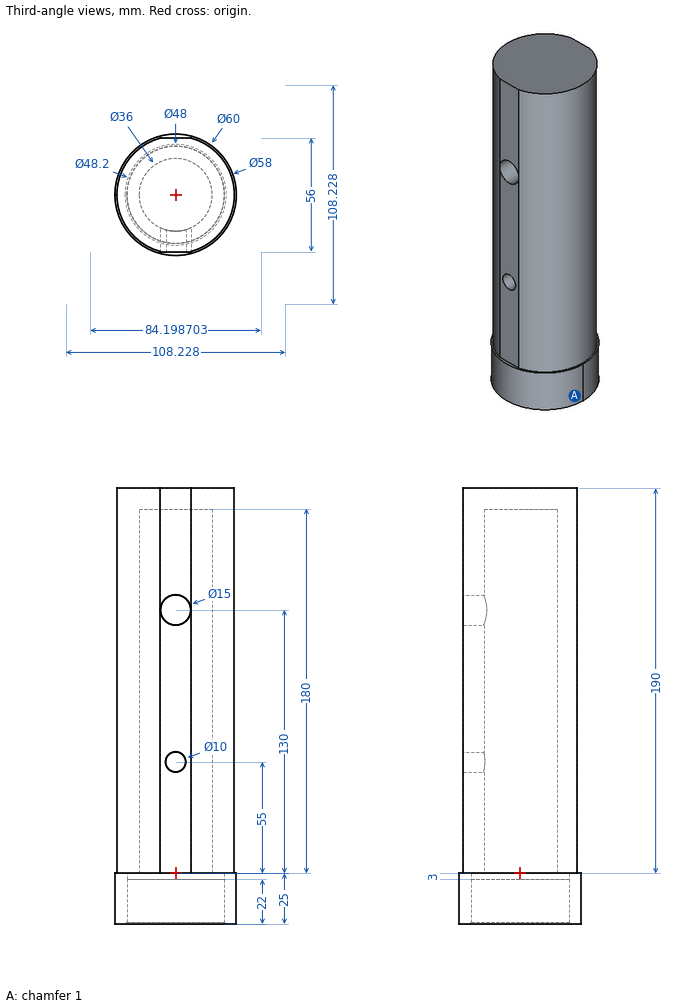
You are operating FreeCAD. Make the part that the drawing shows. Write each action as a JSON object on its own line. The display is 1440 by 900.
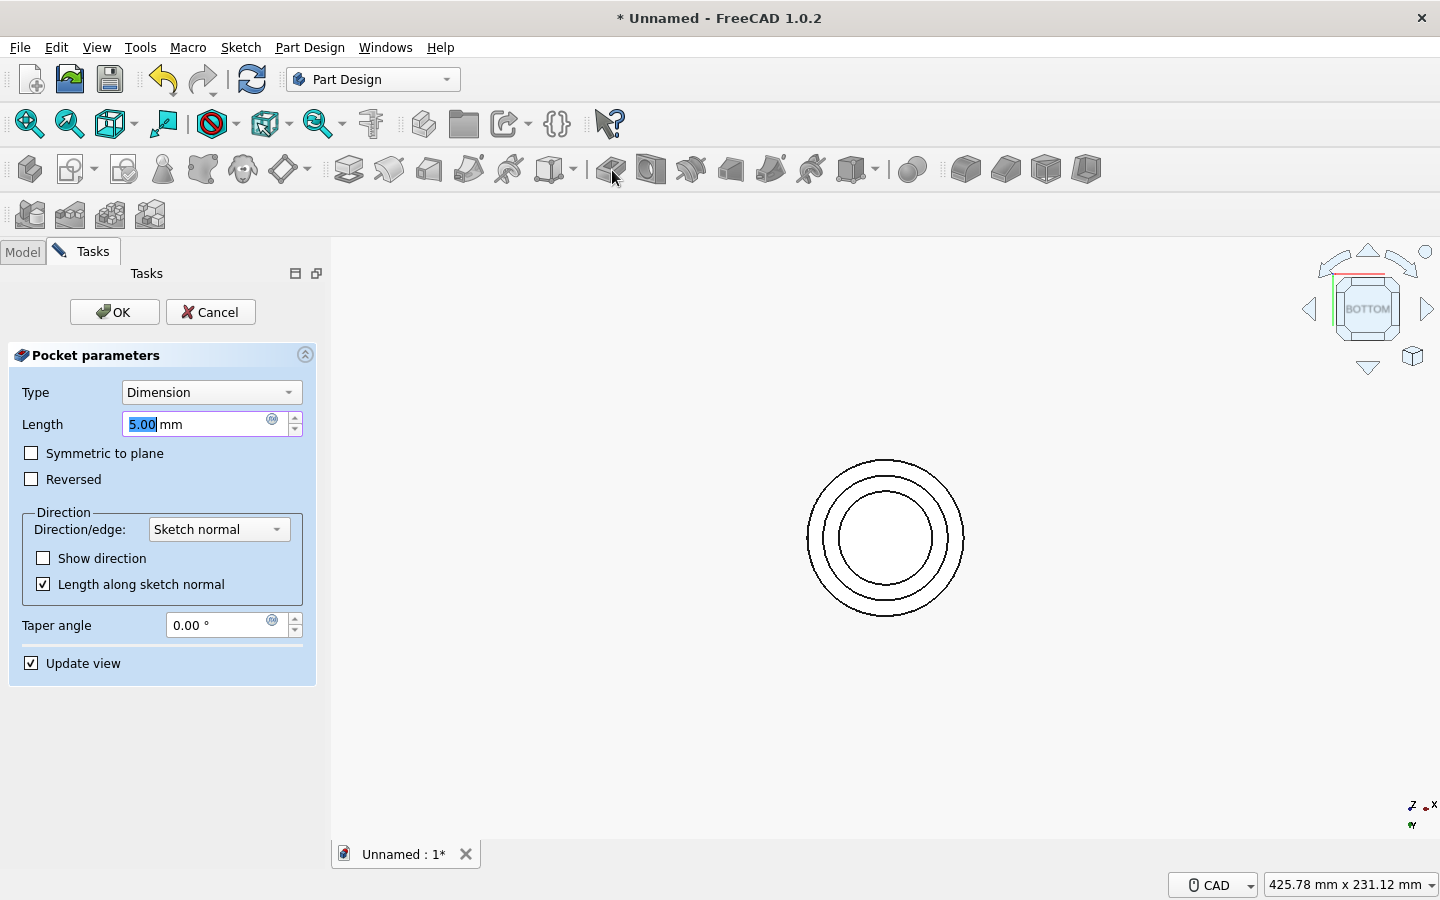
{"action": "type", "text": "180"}
{"action": "key", "text": "Tab"}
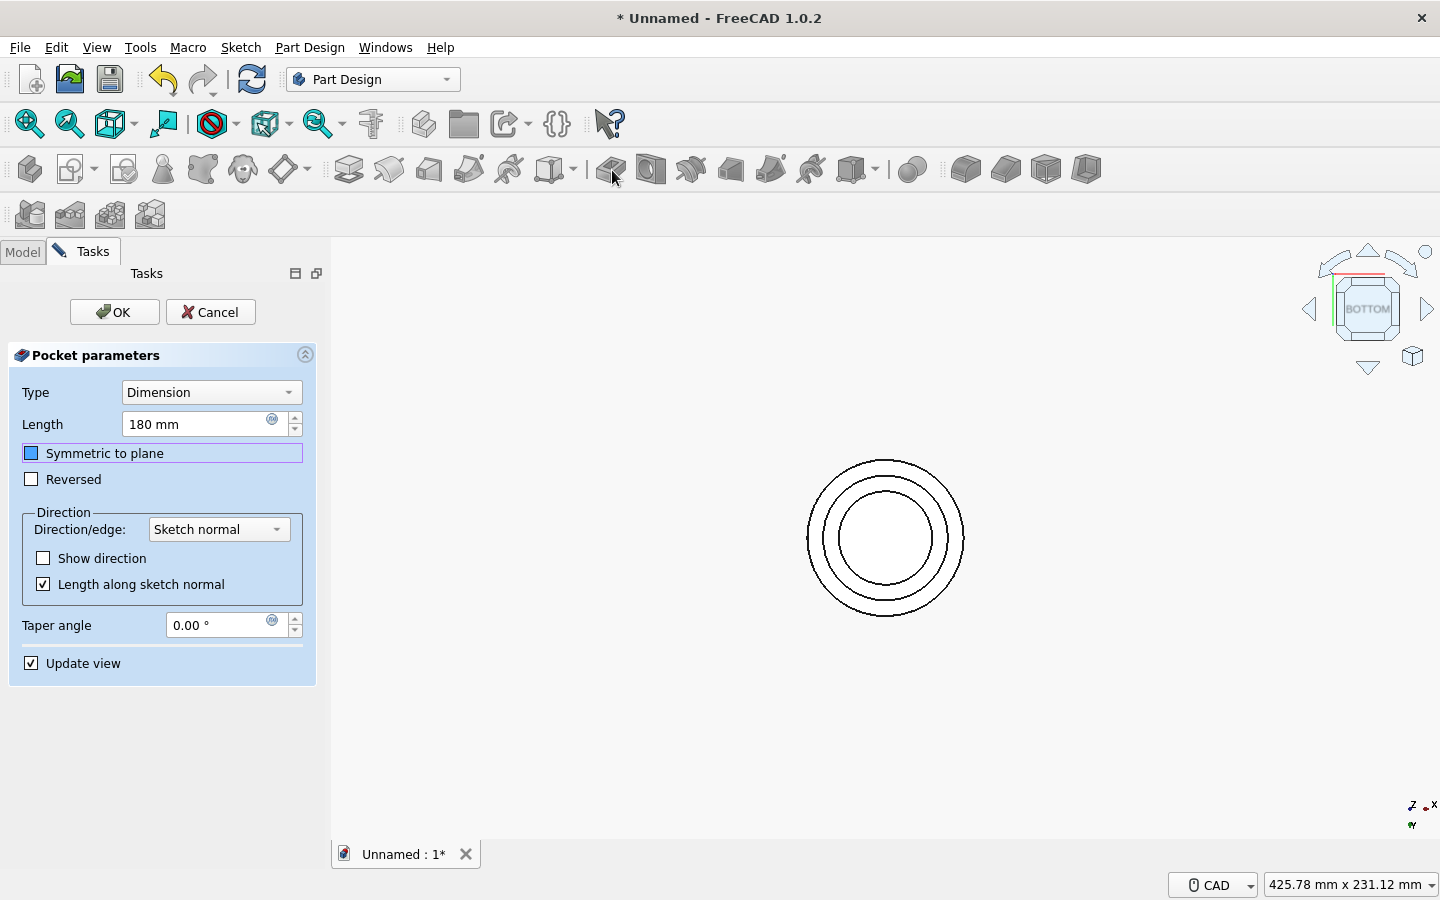
{"action": "left_click", "coordinate": [30, 479]}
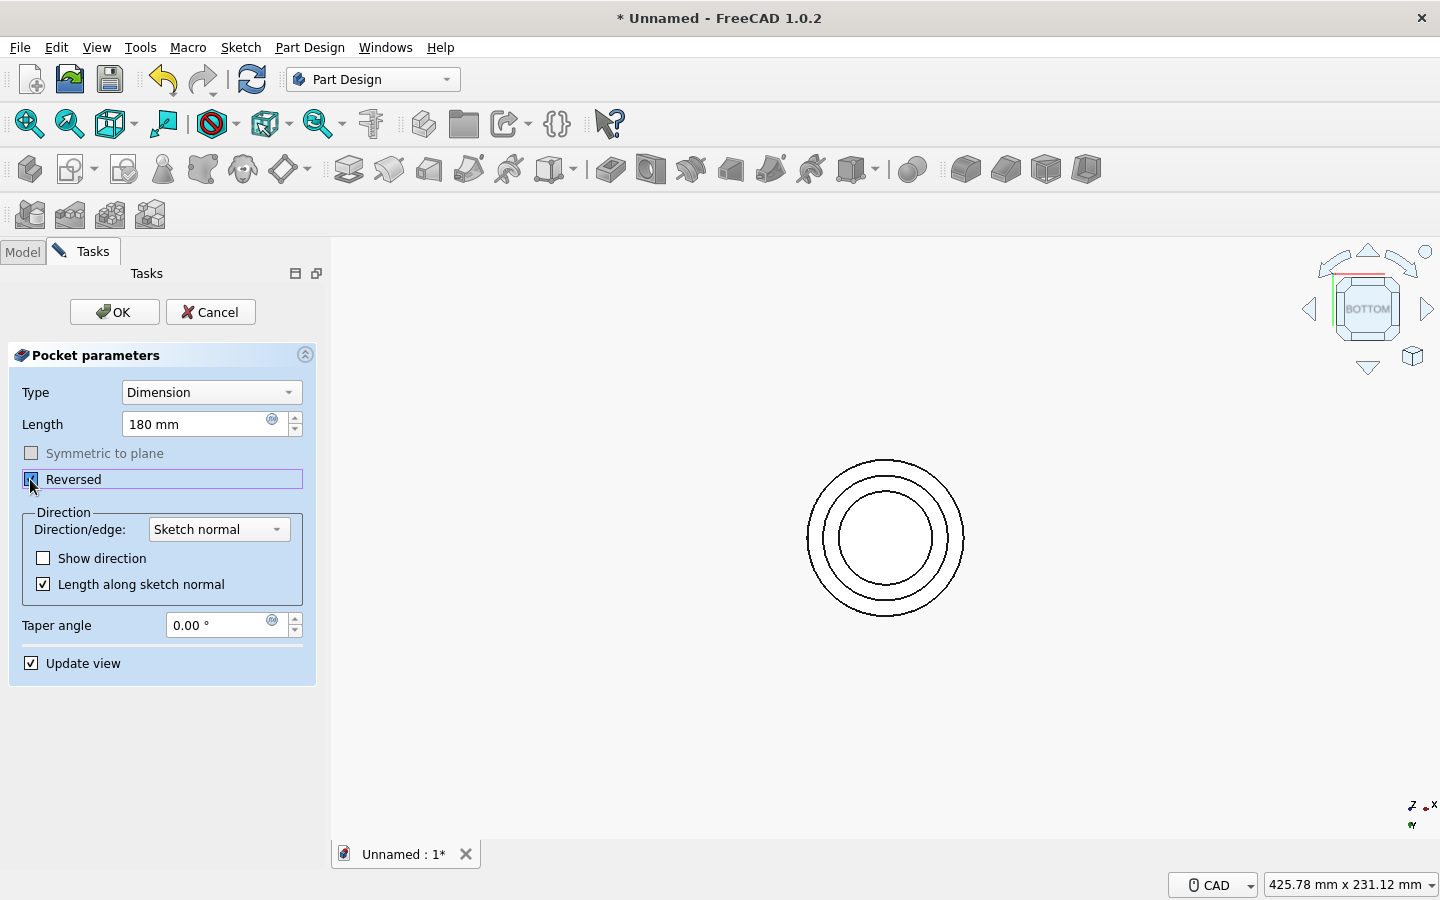
{"action": "left_click", "coordinate": [115, 312]}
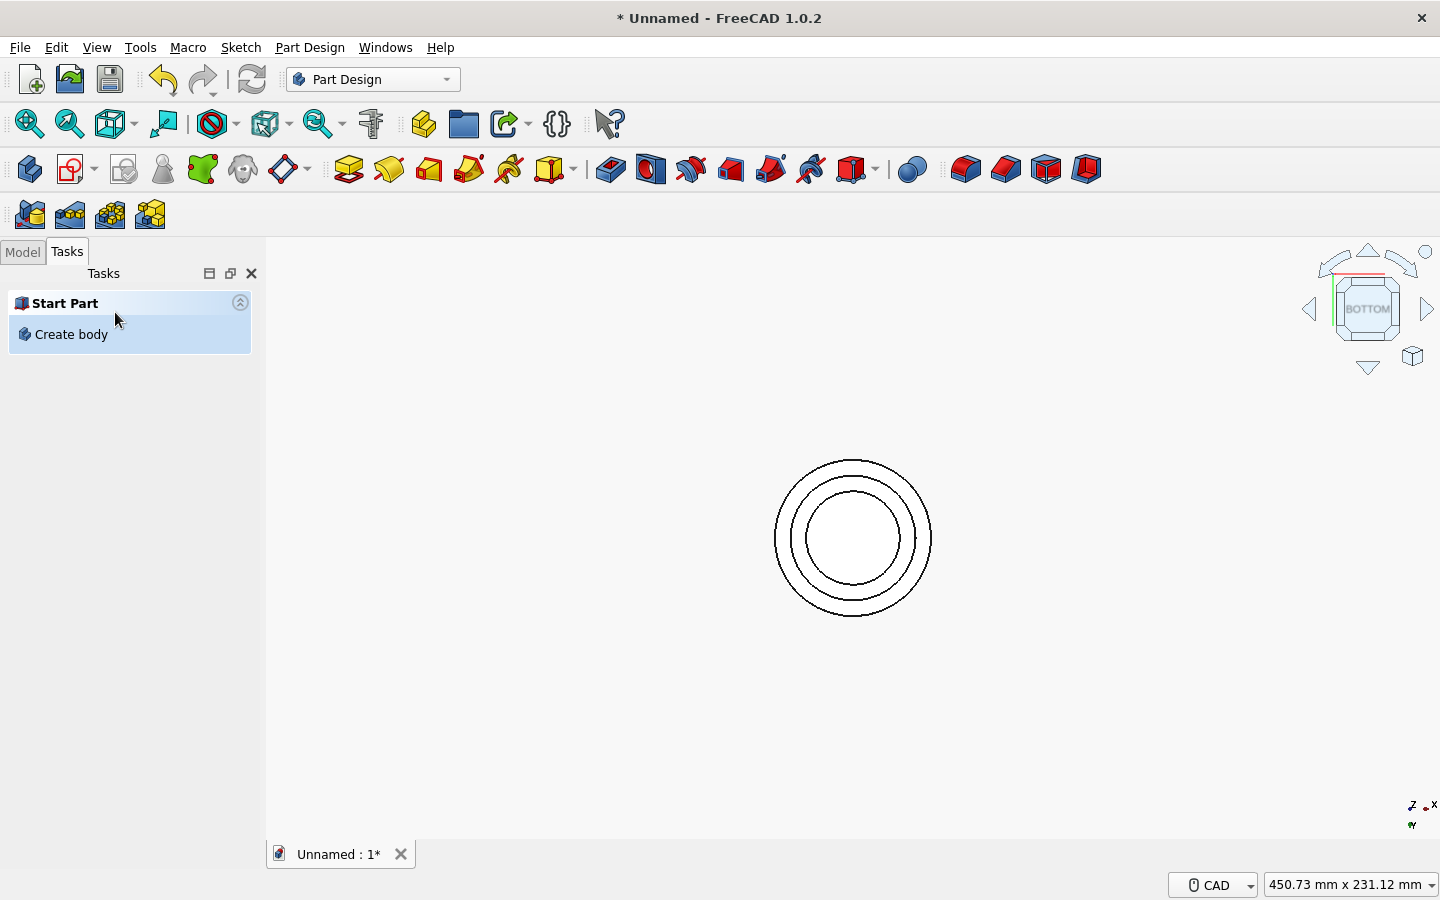
{"action": "left_click", "coordinate": [30, 124]}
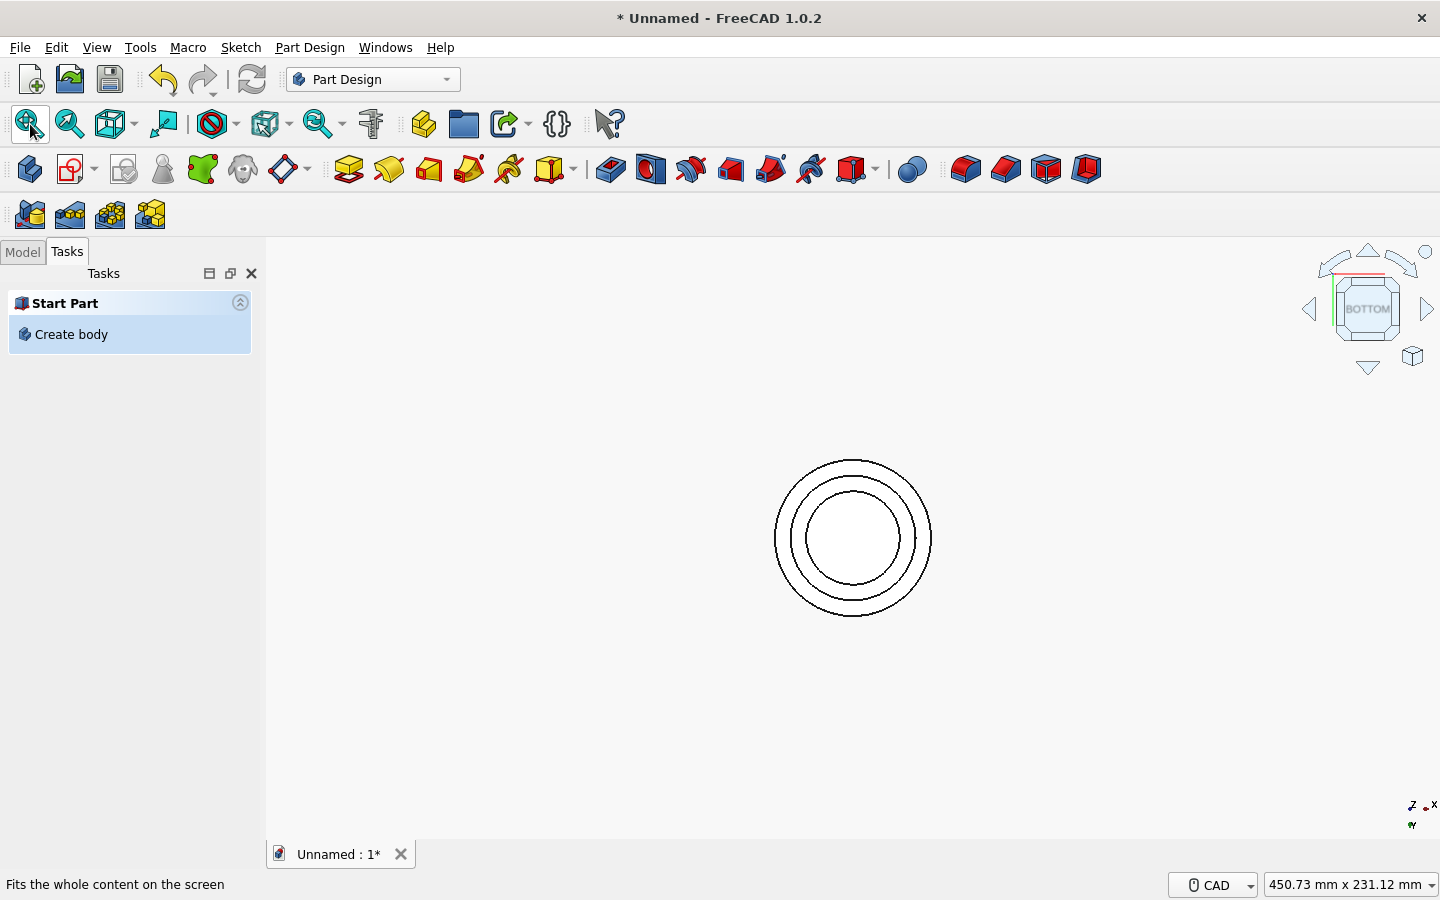
{"action": "left_click", "coordinate": [790, 537]}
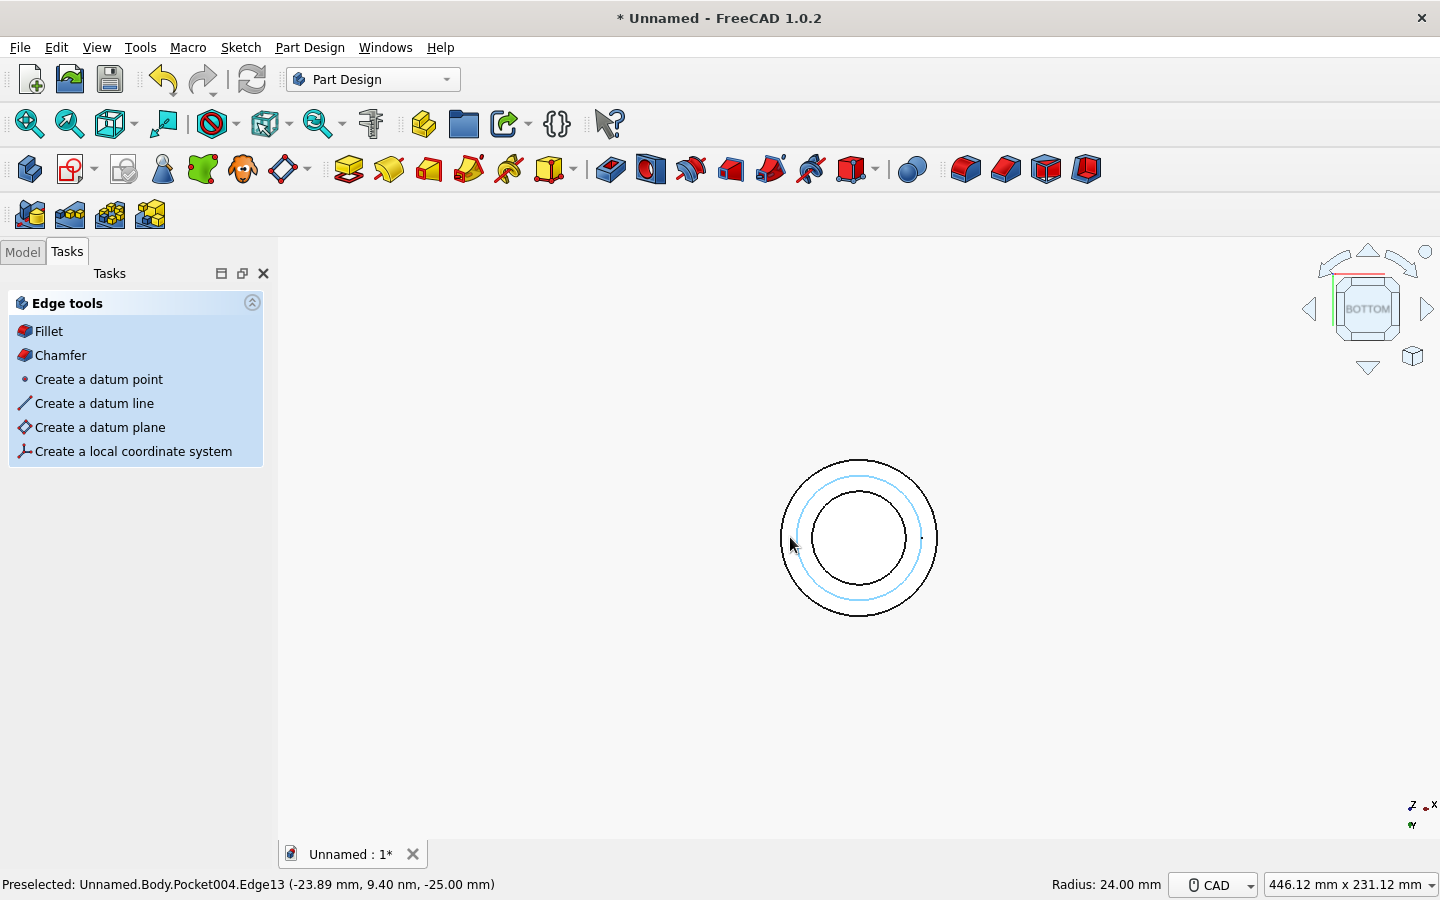
{"action": "left_click", "coordinate": [1006, 170]}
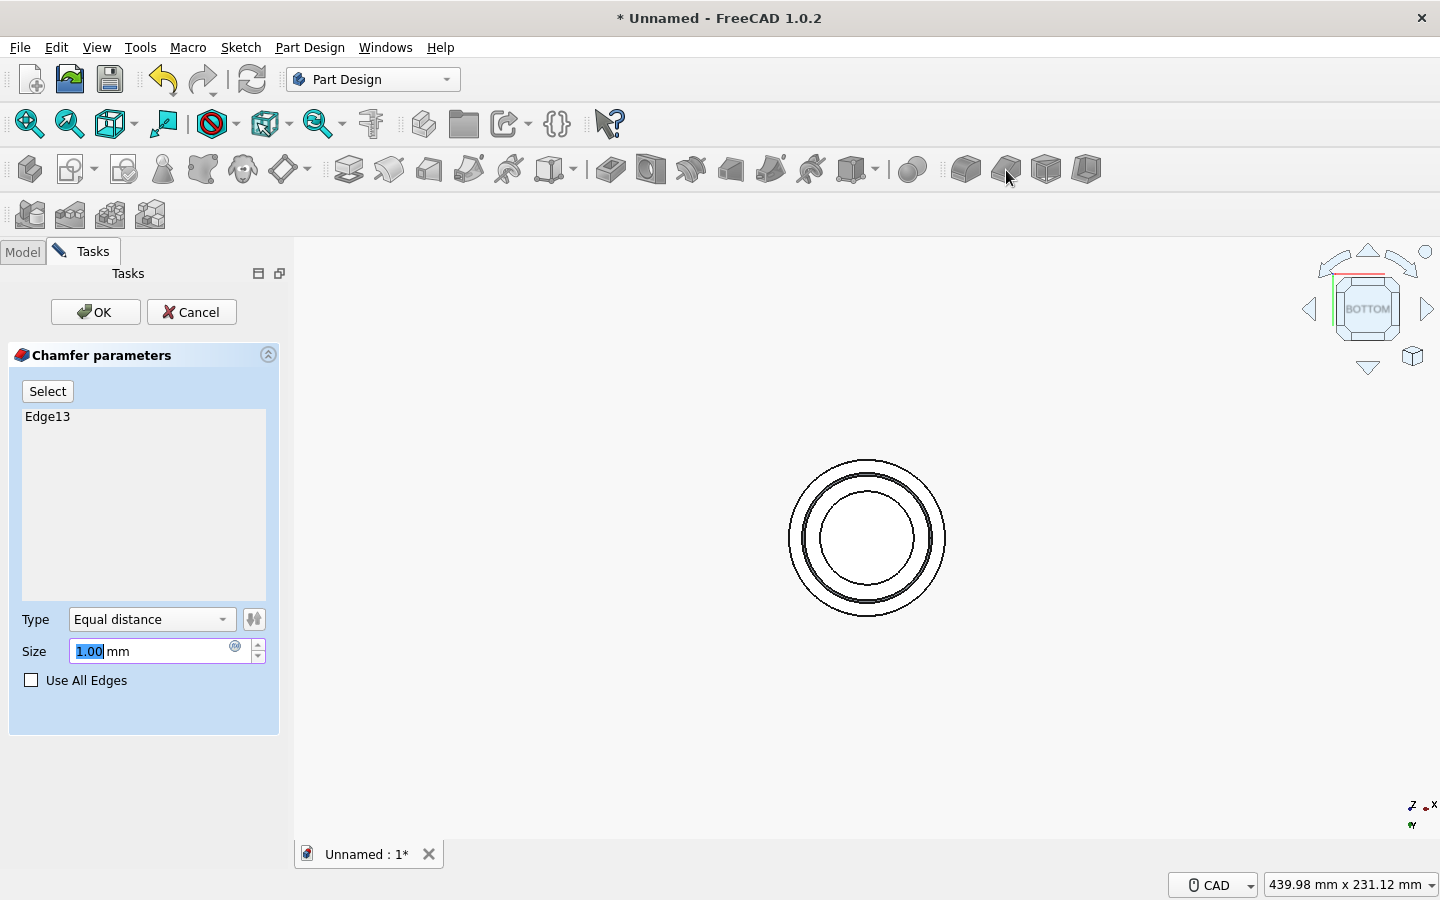
{"action": "type", "text": "1"}
{"action": "key", "text": "Tab"}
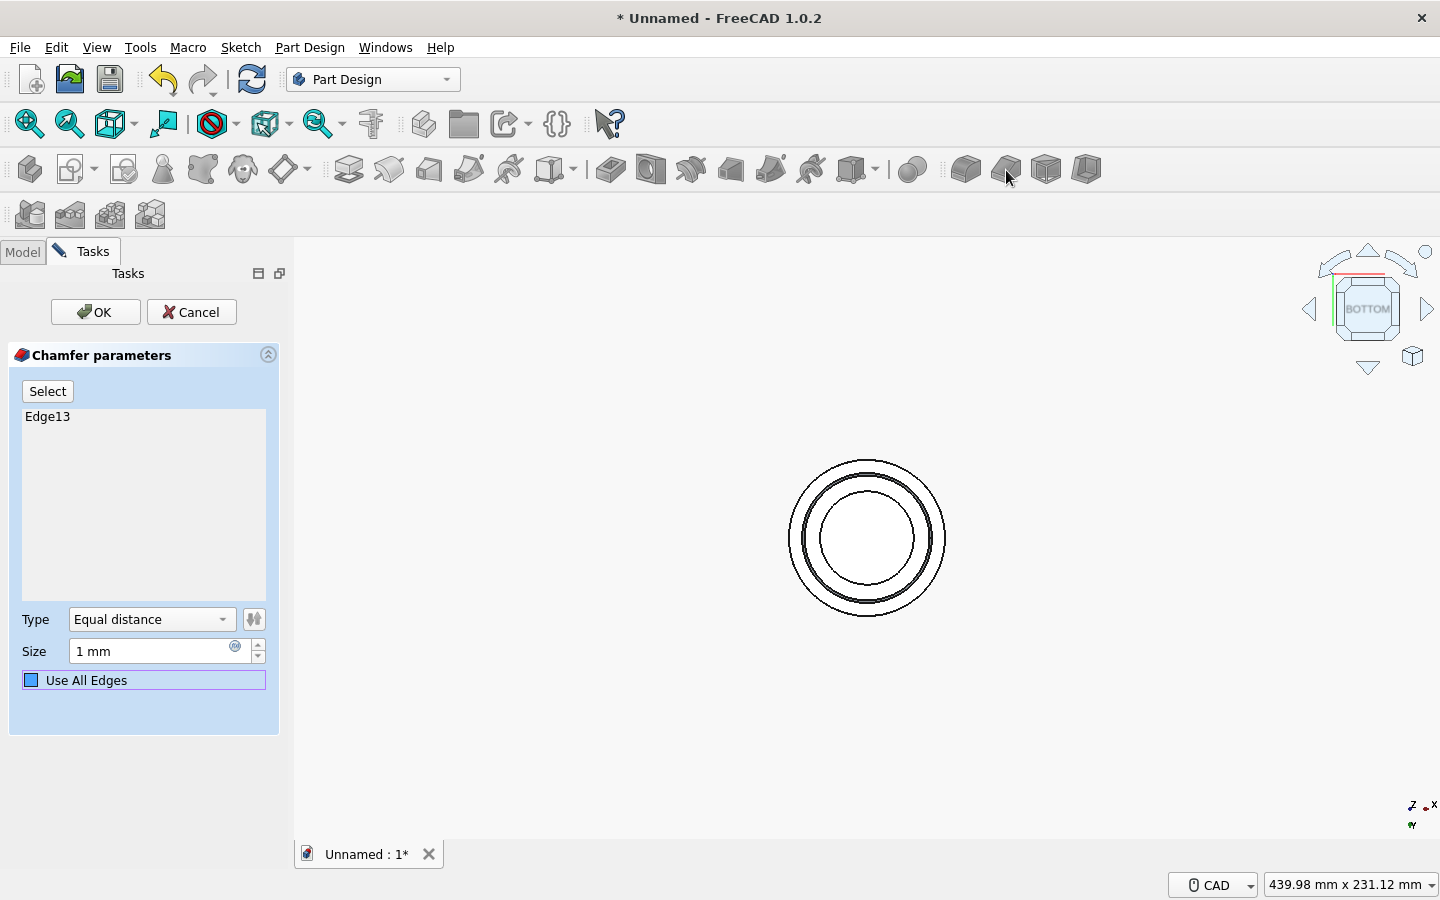
{"action": "left_click", "coordinate": [96, 312]}